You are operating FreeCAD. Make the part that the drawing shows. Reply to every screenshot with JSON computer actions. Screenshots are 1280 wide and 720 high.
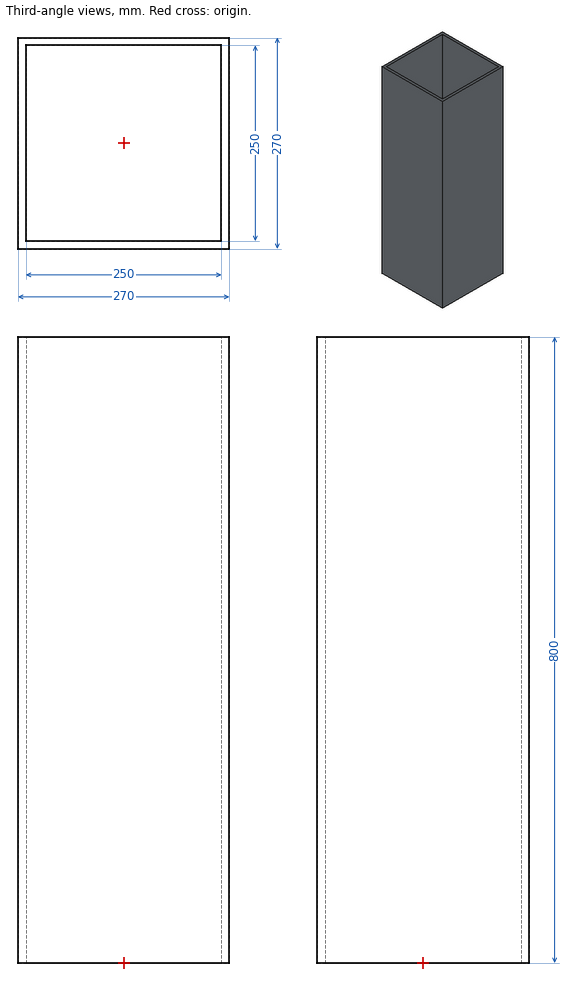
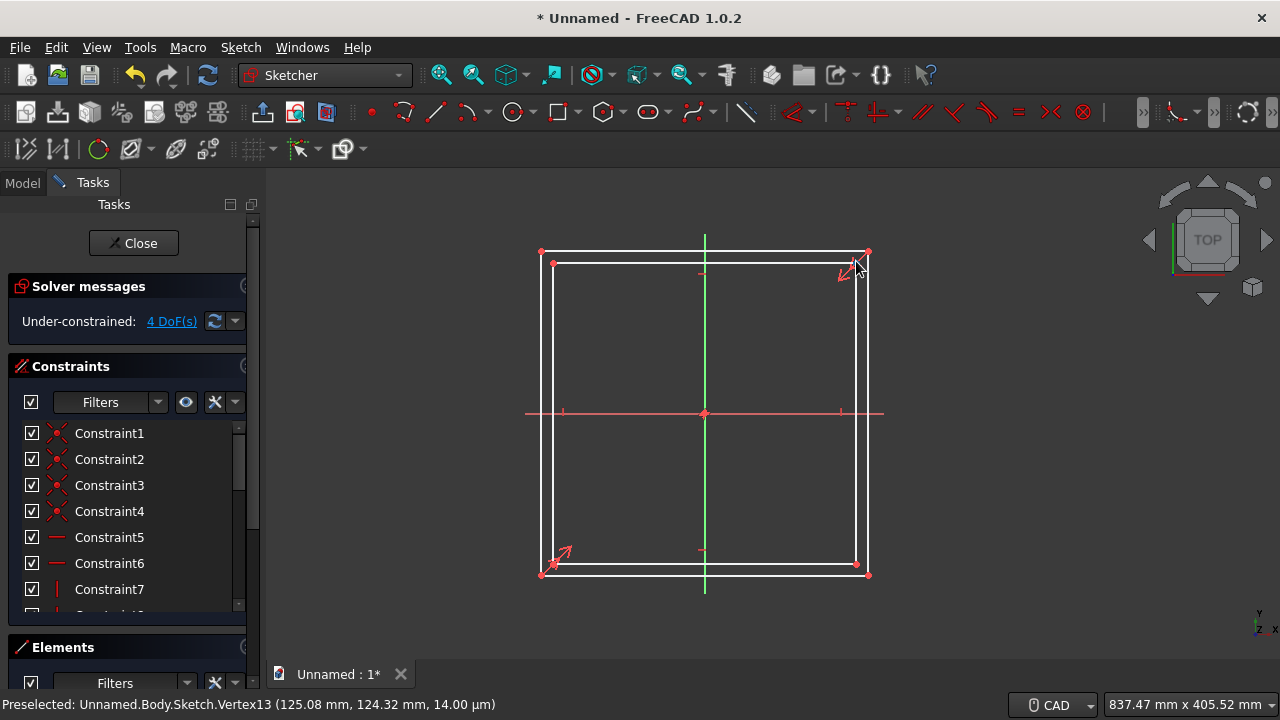
{"action": "left_click", "coordinate": [639, 576]}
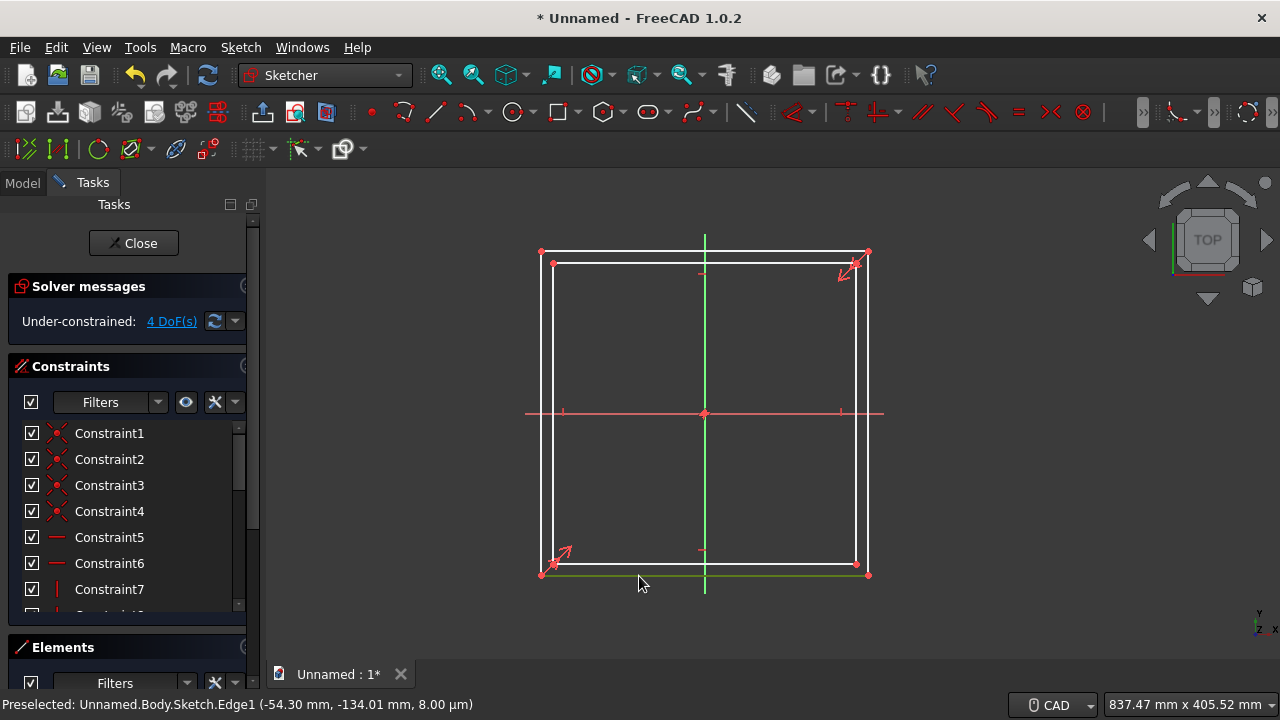
{"action": "key", "text": "l"}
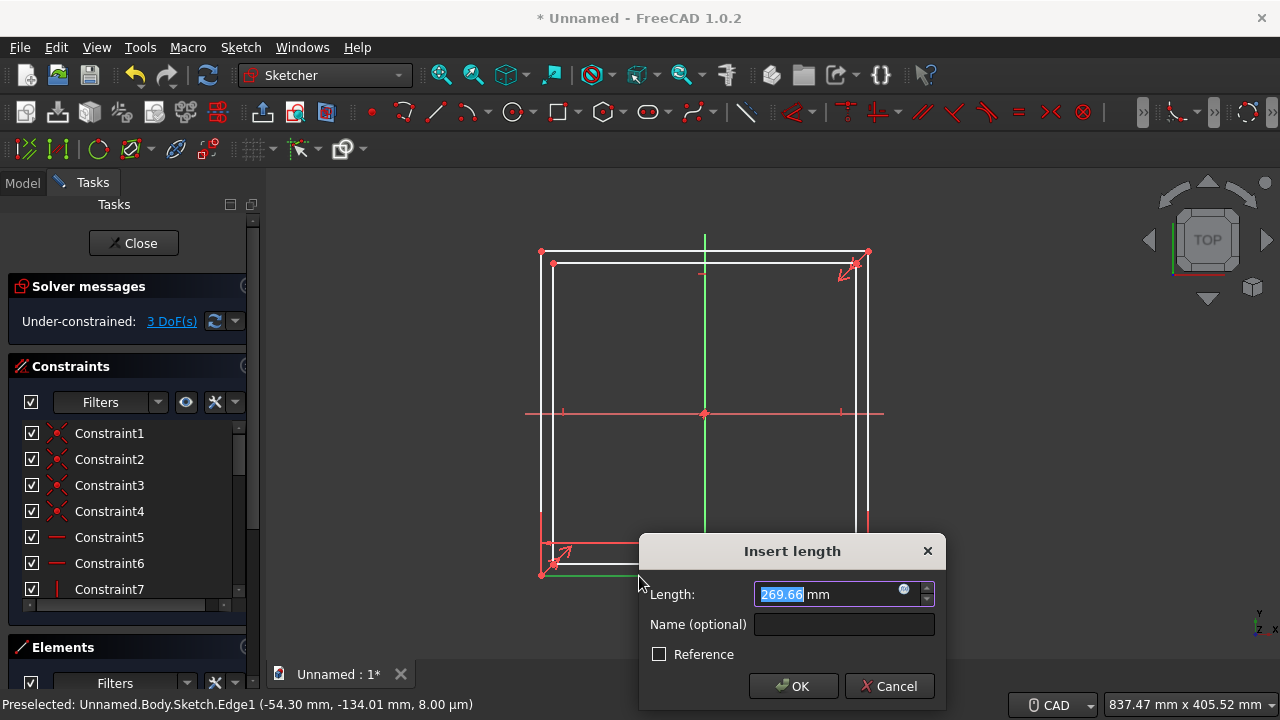
{"action": "type", "text": "270"}
{"action": "key", "text": "Return"}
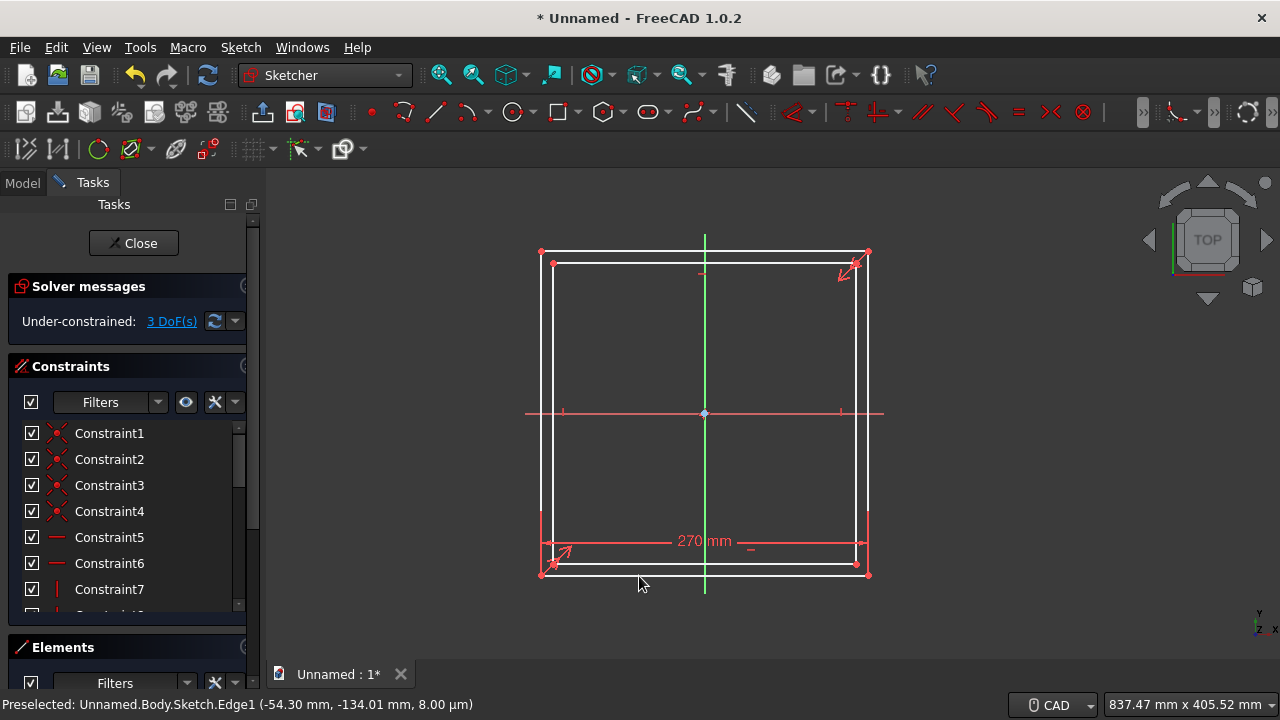
{"action": "left_click", "coordinate": [868, 478]}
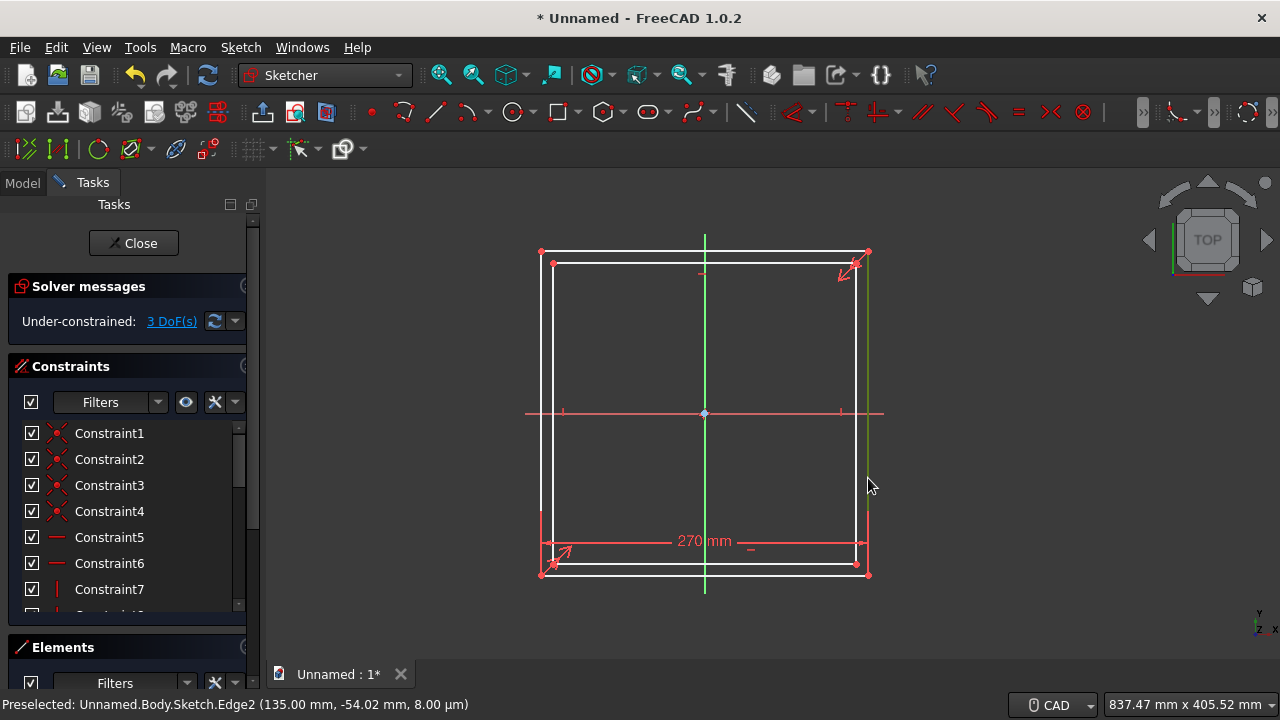
{"action": "left_click", "coordinate": [814, 112]}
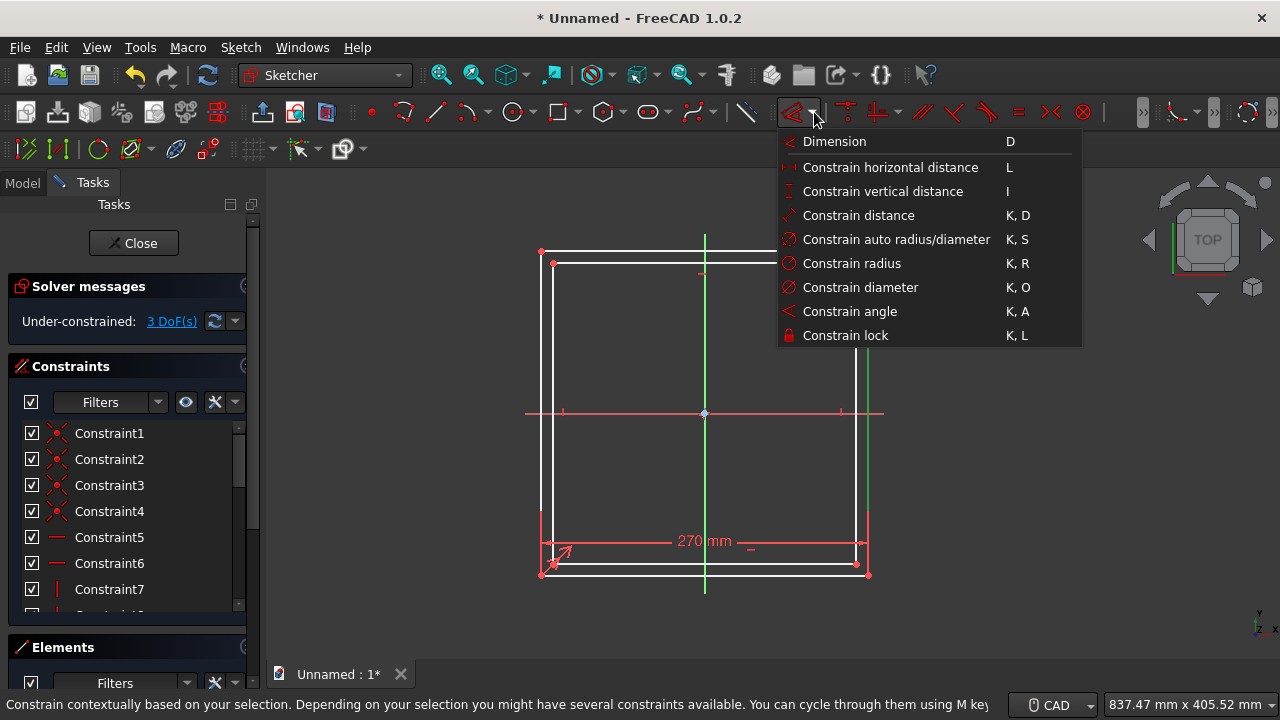
{"action": "left_click", "coordinate": [930, 191]}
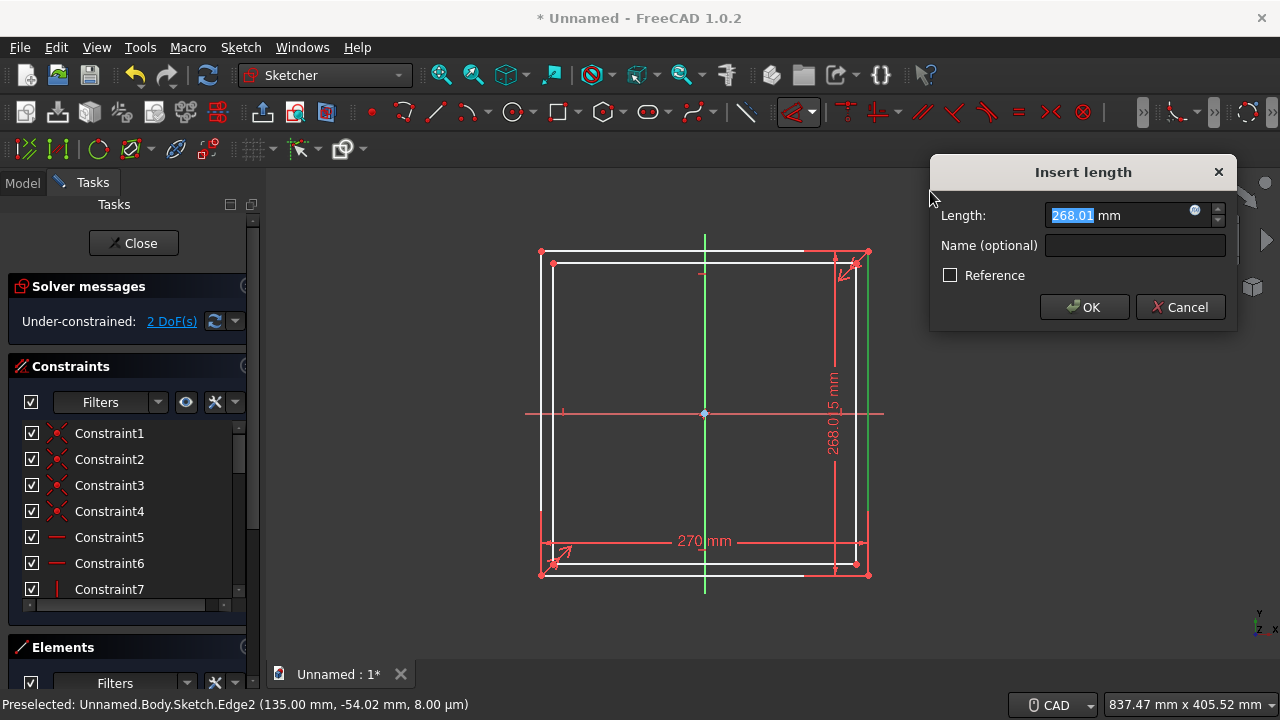
{"action": "type", "text": "270"}
{"action": "key", "text": "Return"}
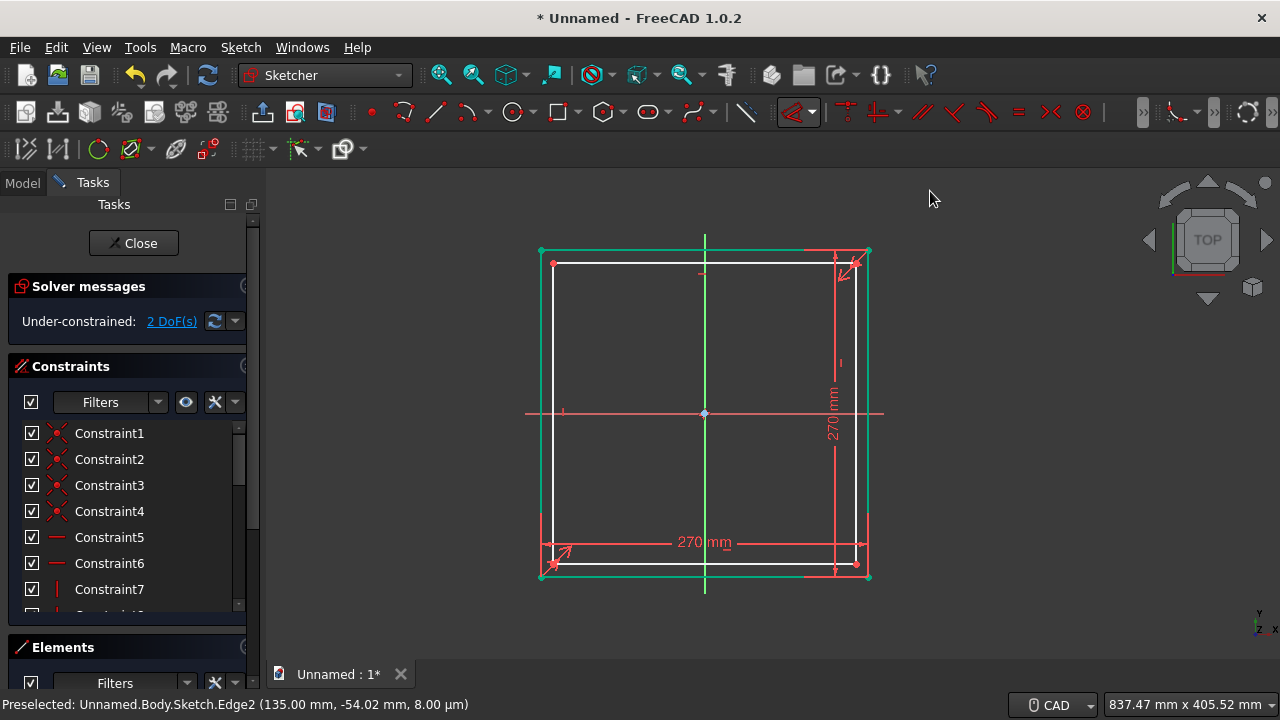
{"action": "left_click", "coordinate": [644, 564]}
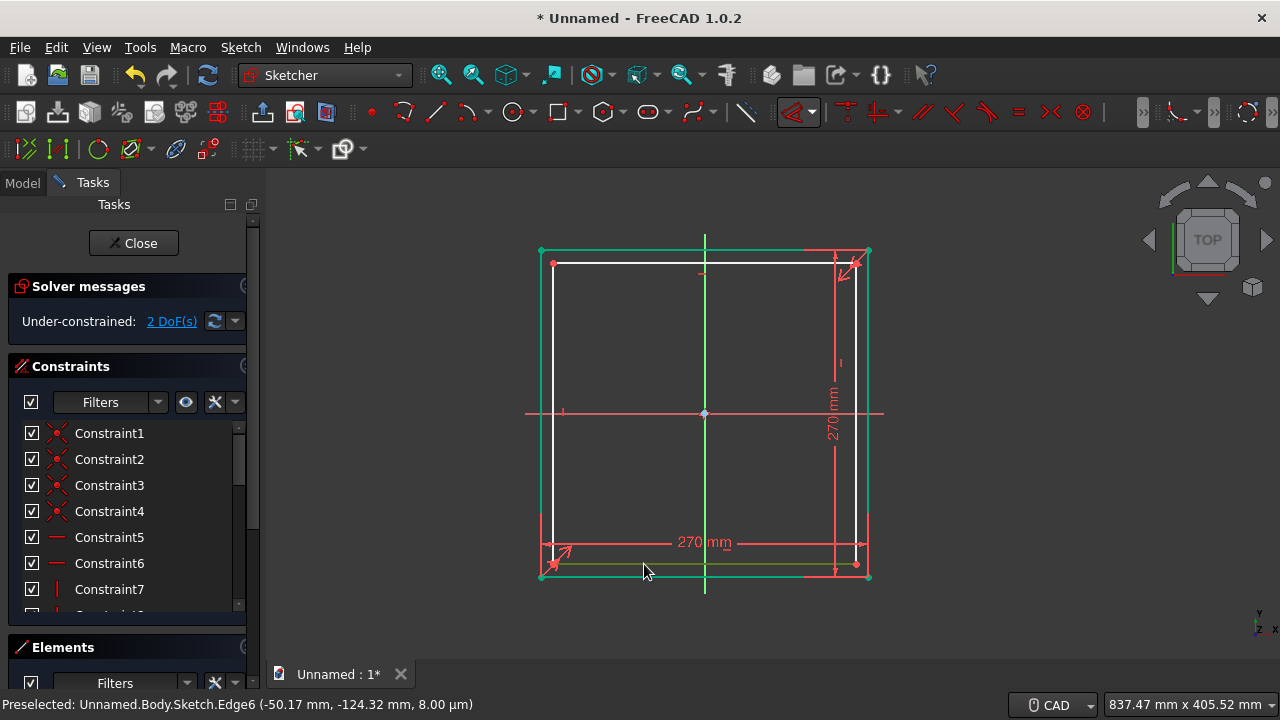
{"action": "key", "text": "l"}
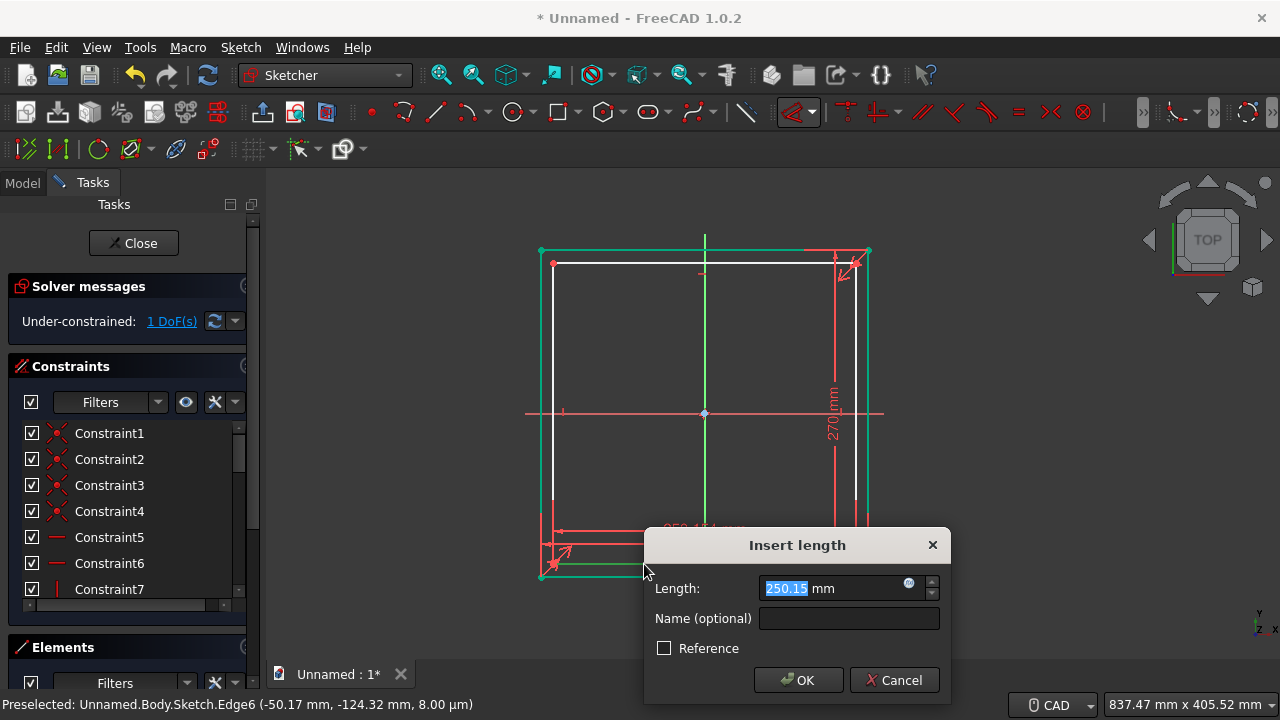
{"action": "type", "text": "250"}
{"action": "key", "text": "Return"}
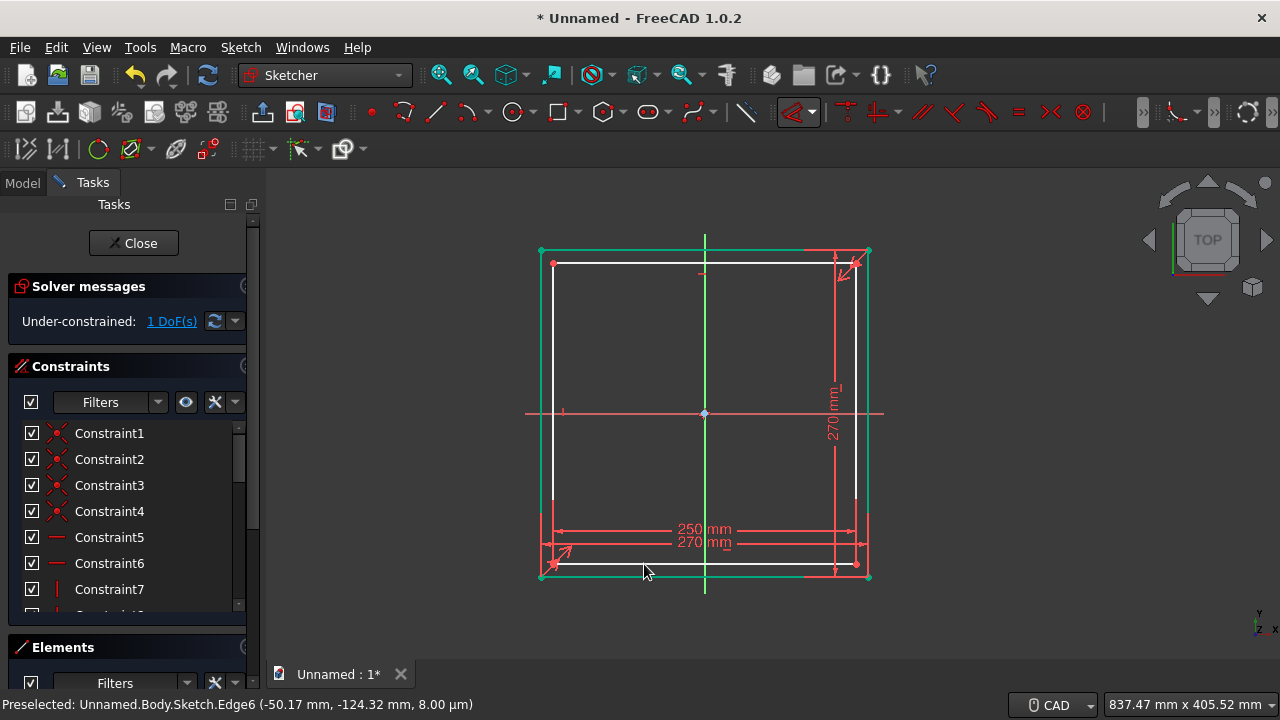
{"action": "left_click", "coordinate": [856, 474]}